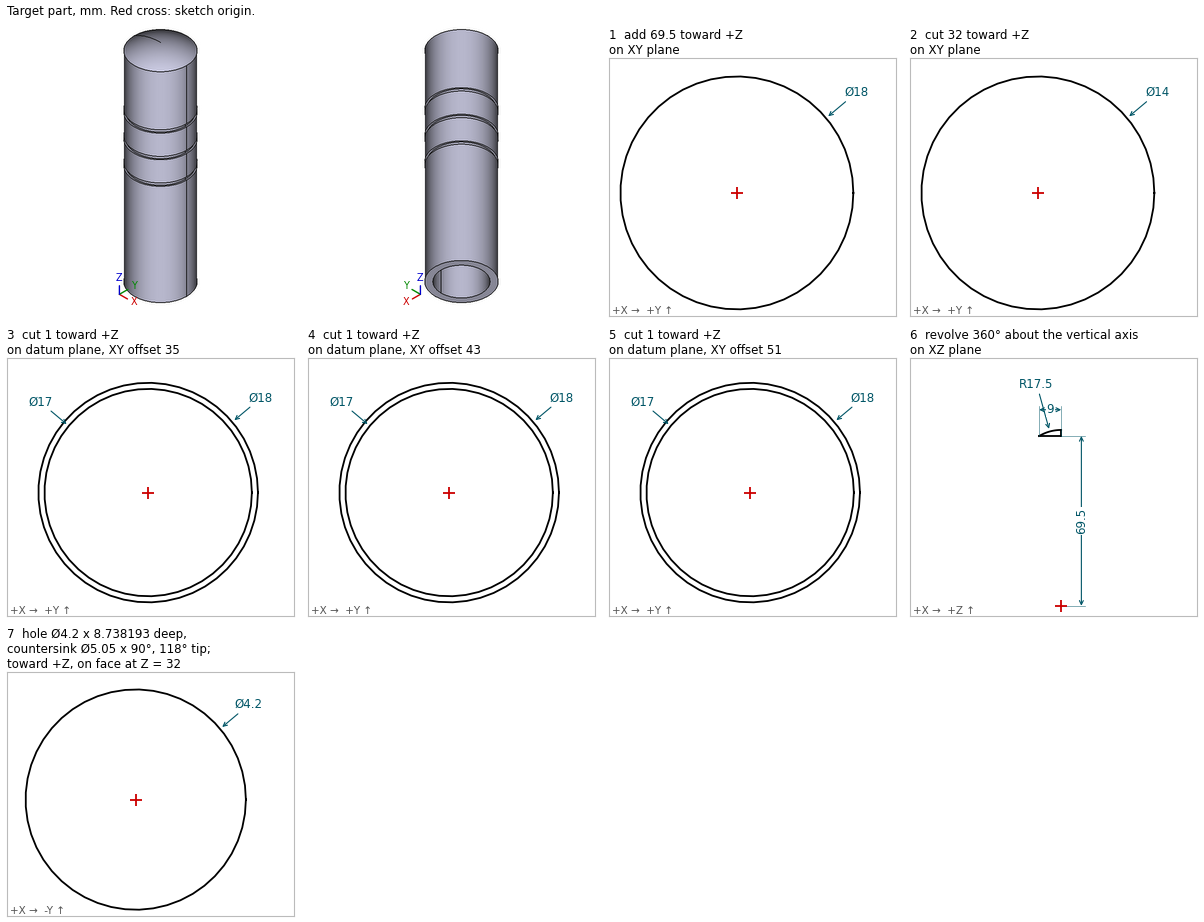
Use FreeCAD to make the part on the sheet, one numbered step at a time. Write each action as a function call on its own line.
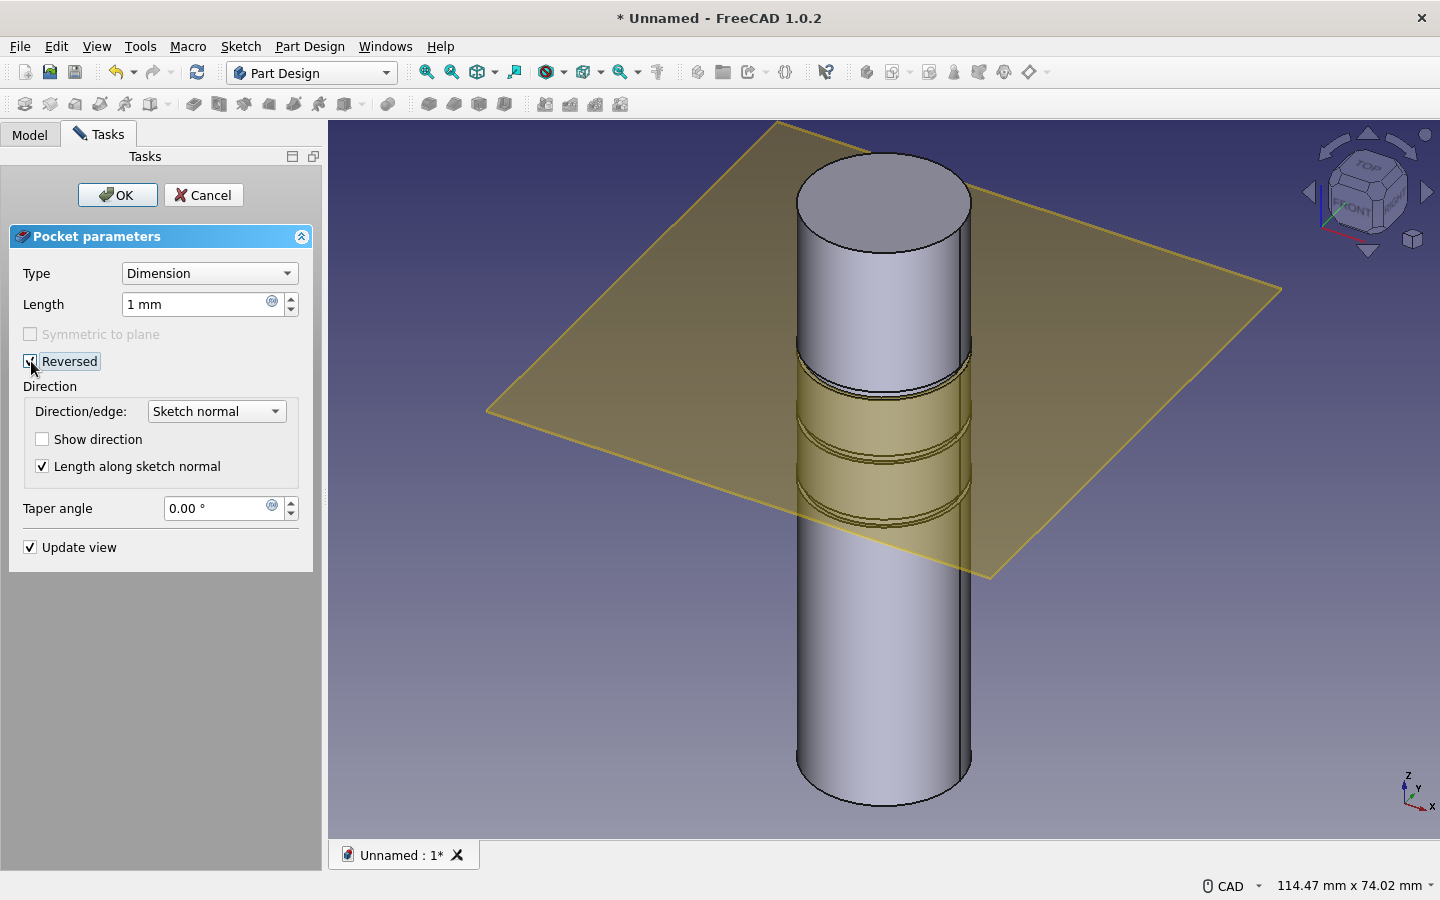
click(118, 195)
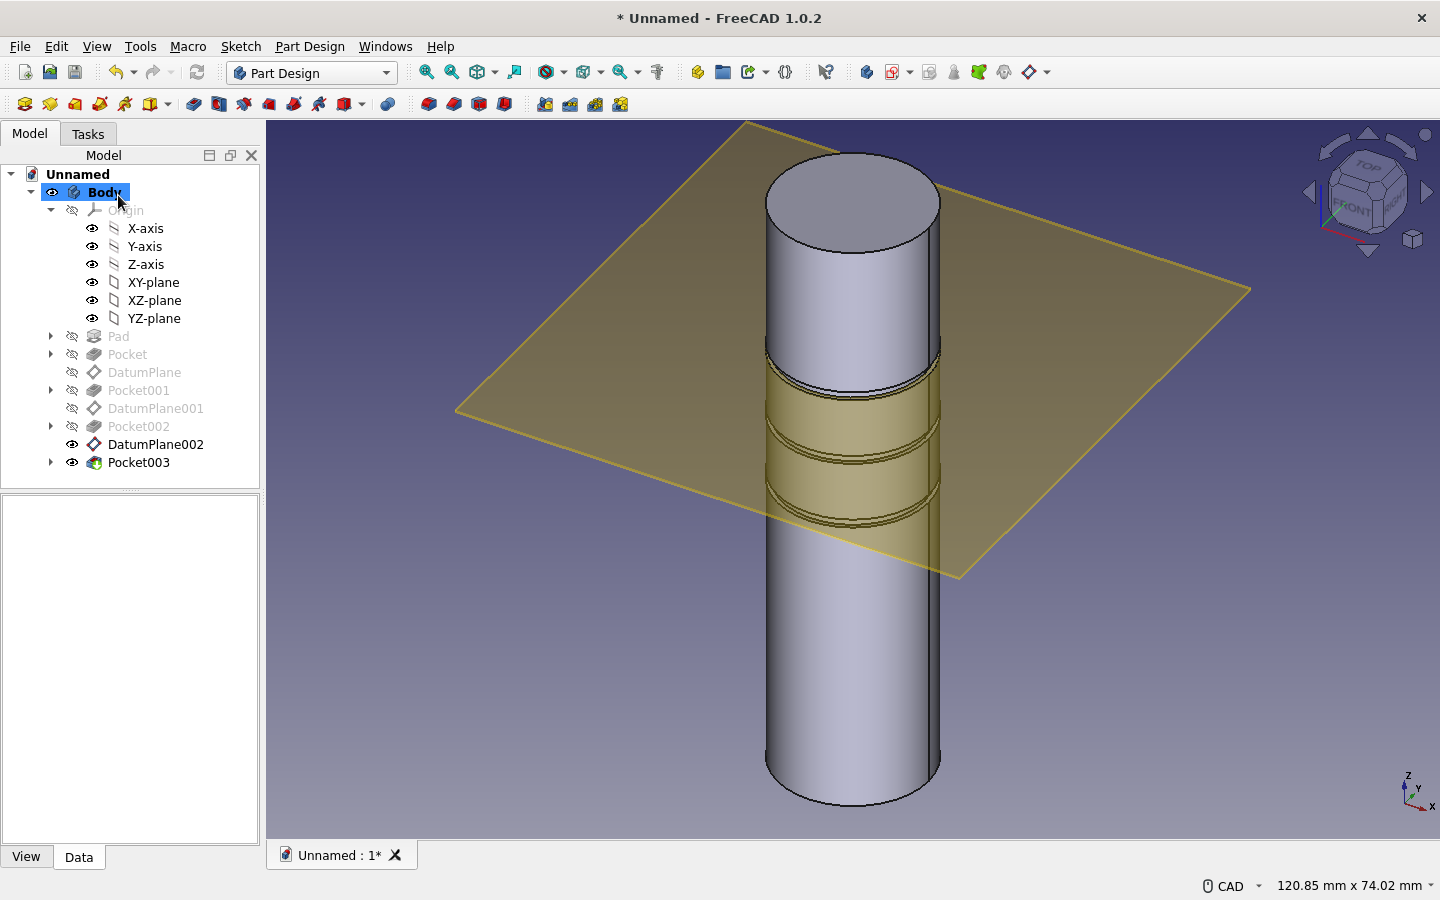
click(117, 444)
key(space)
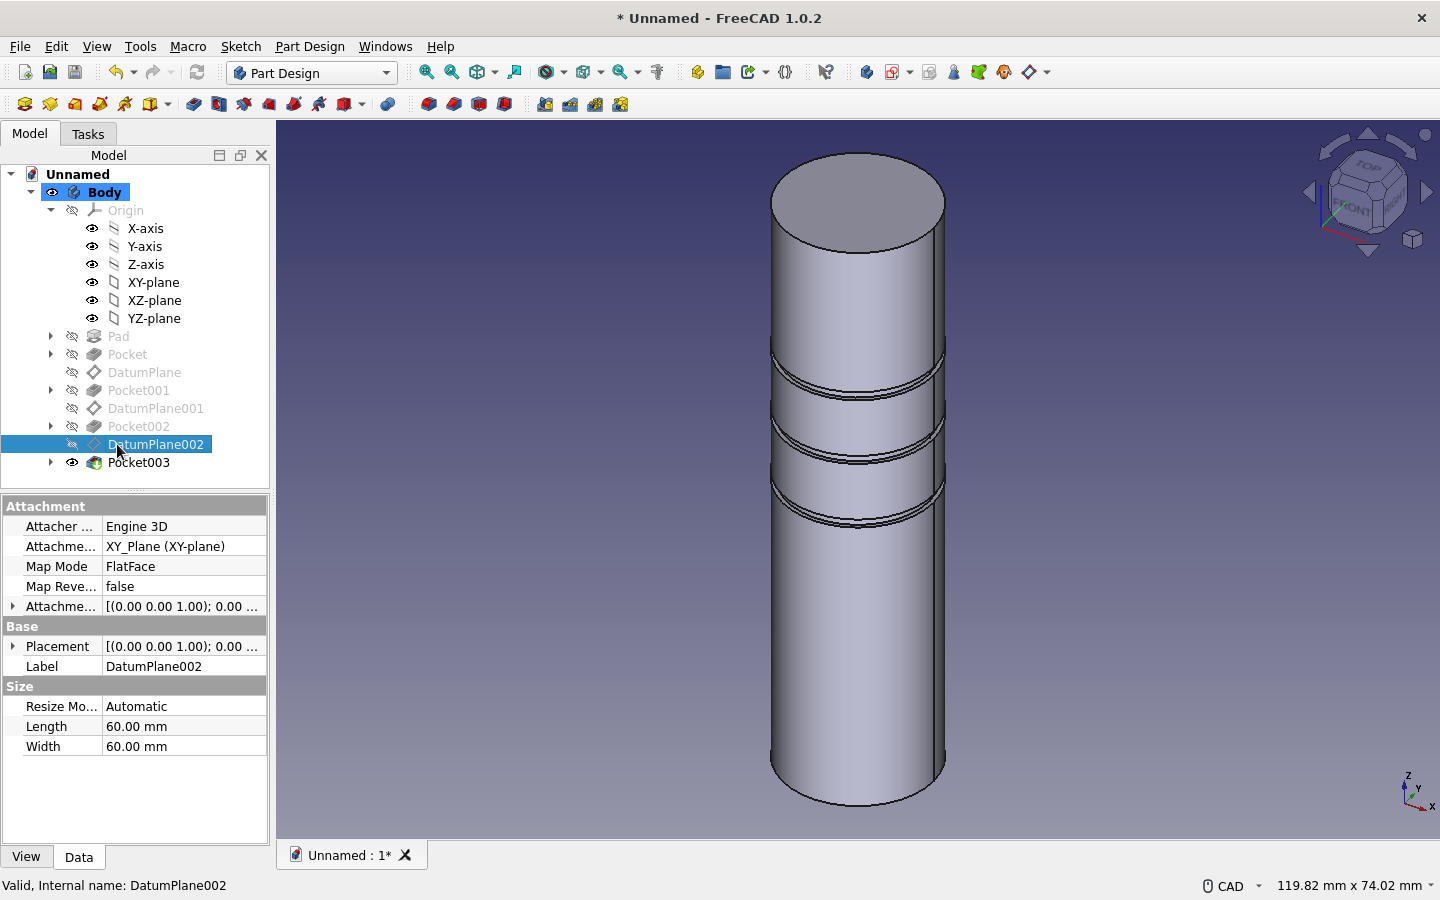
click(316, 799)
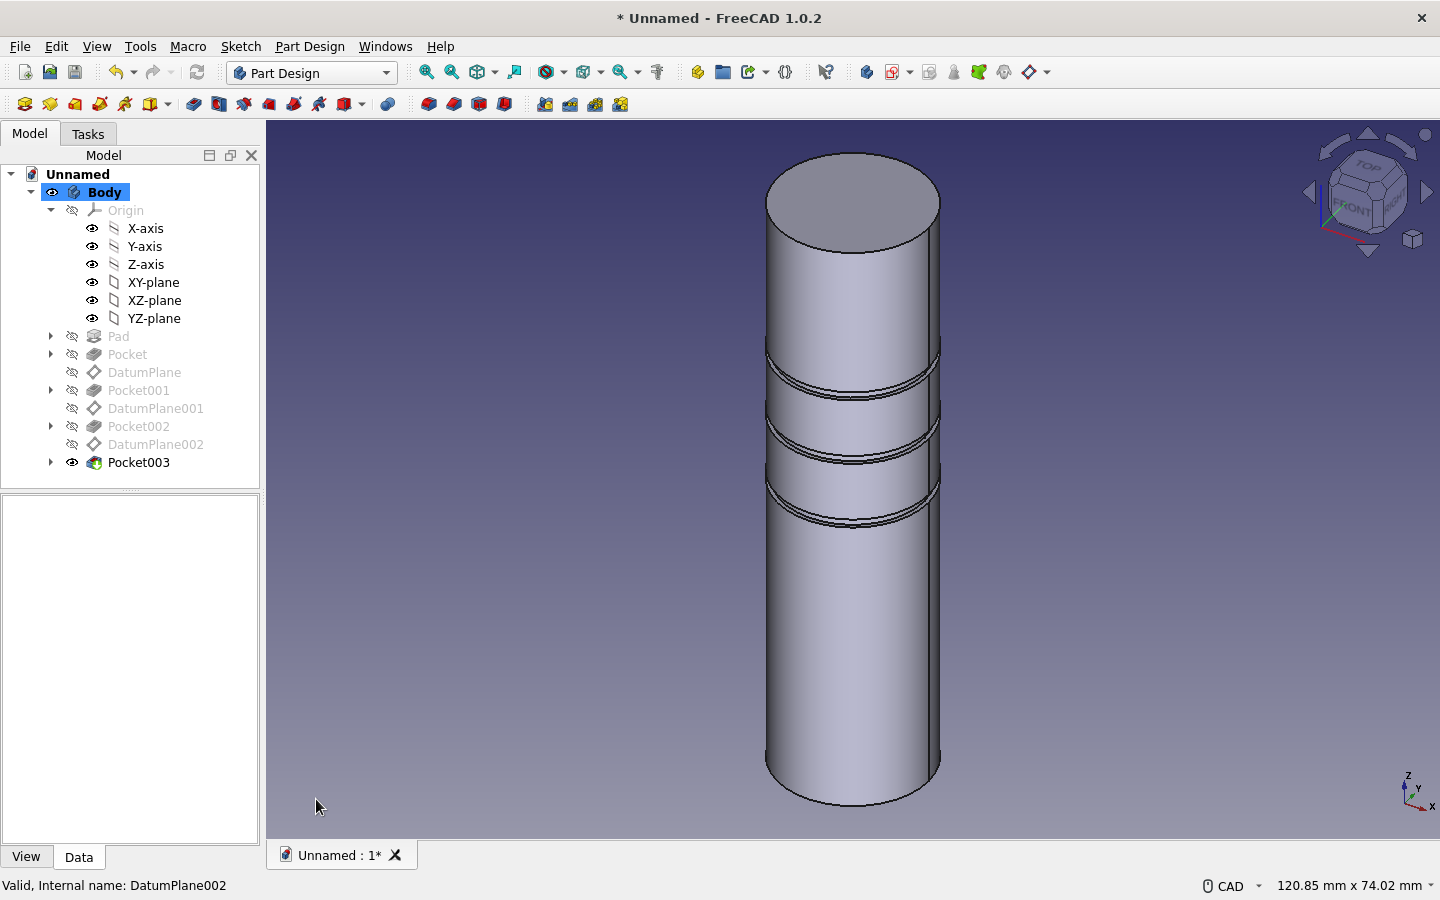
click(892, 72)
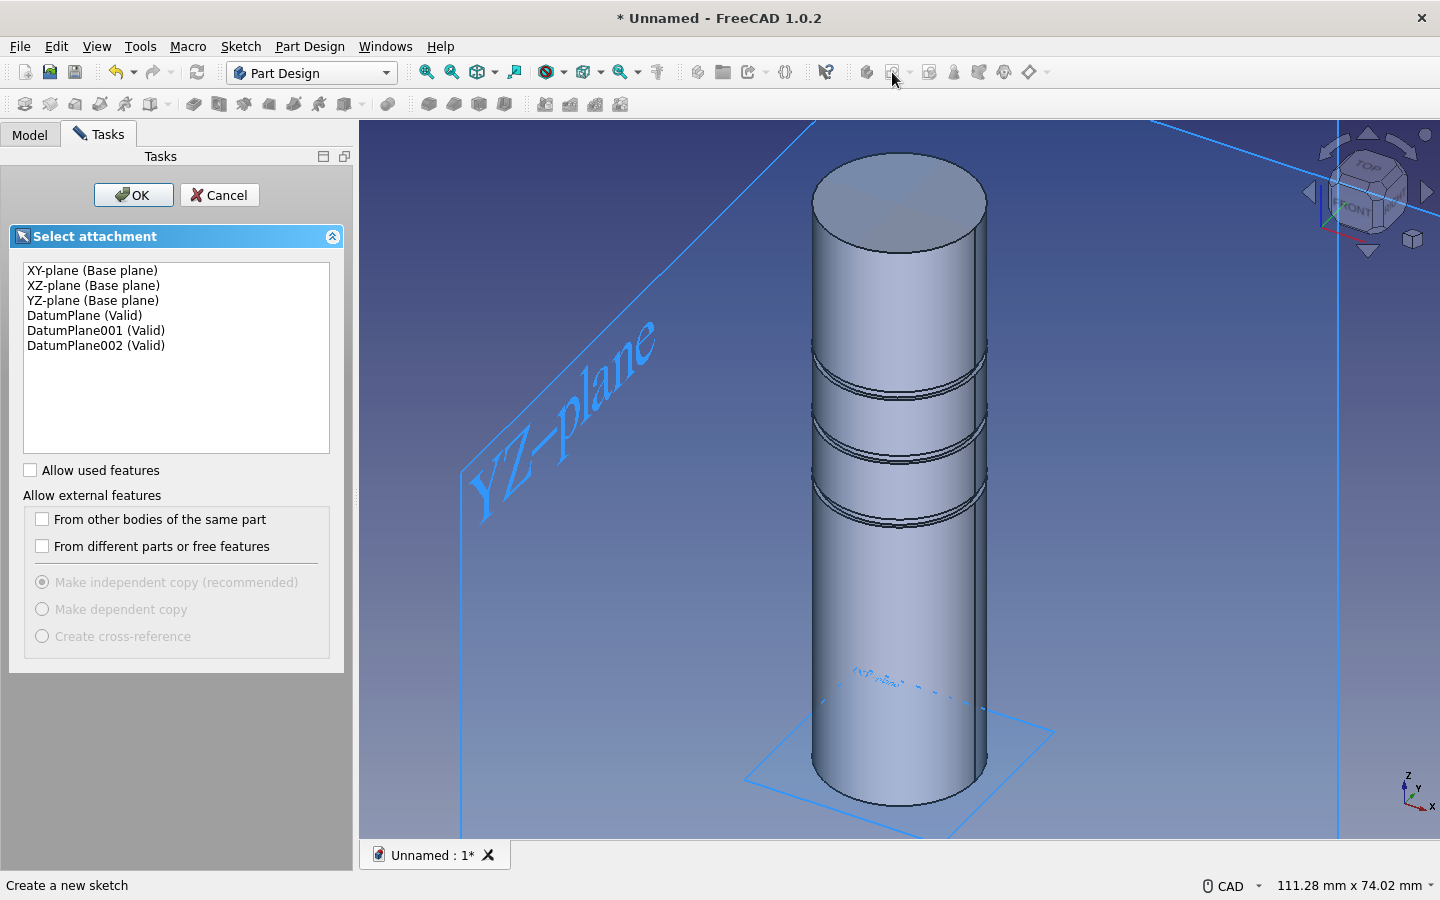
click(84, 286)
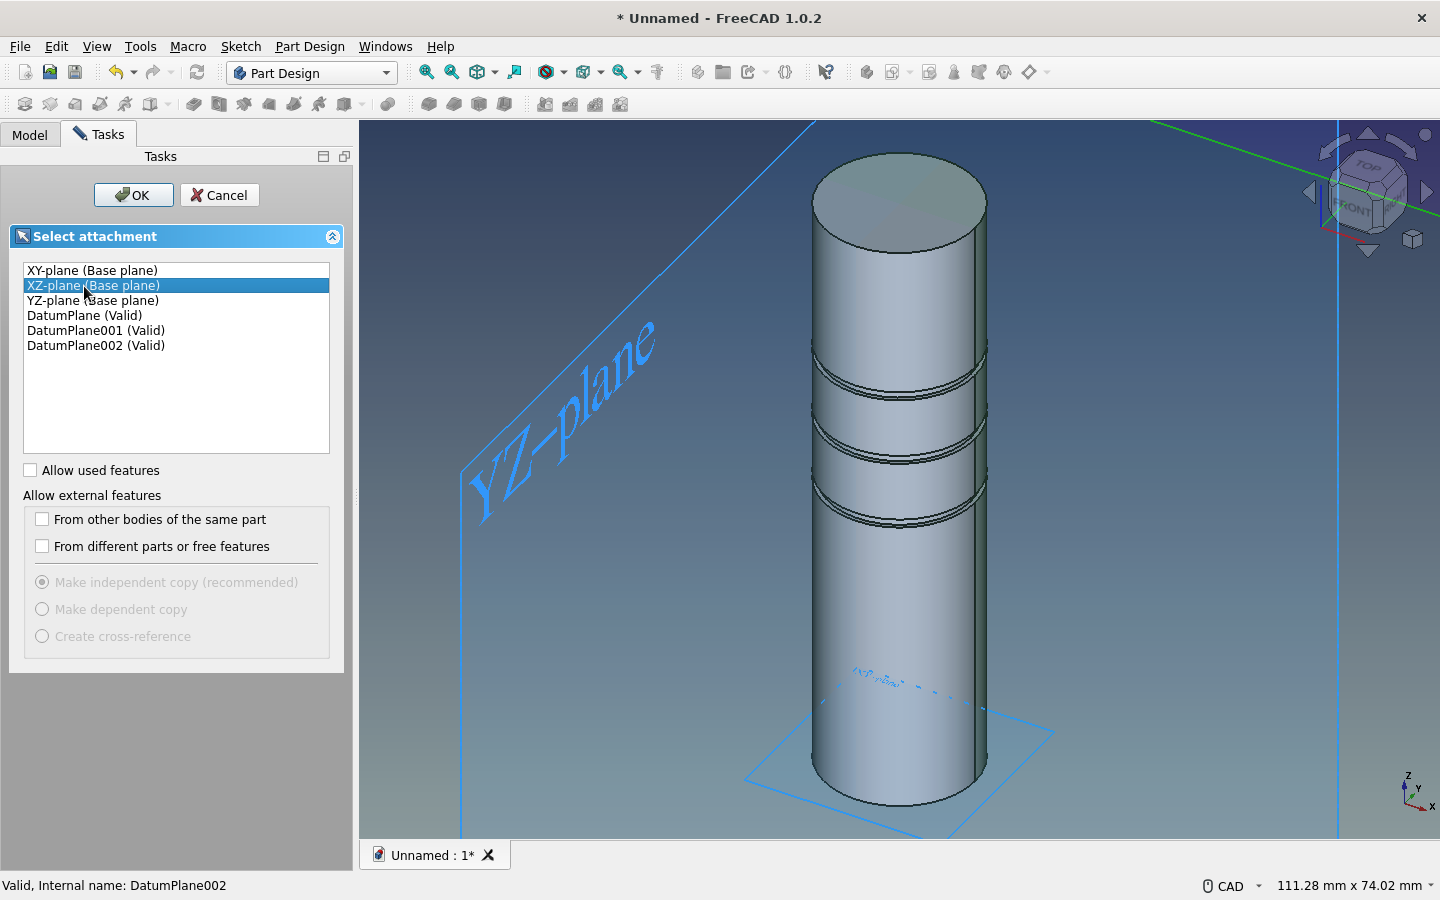
click(134, 195)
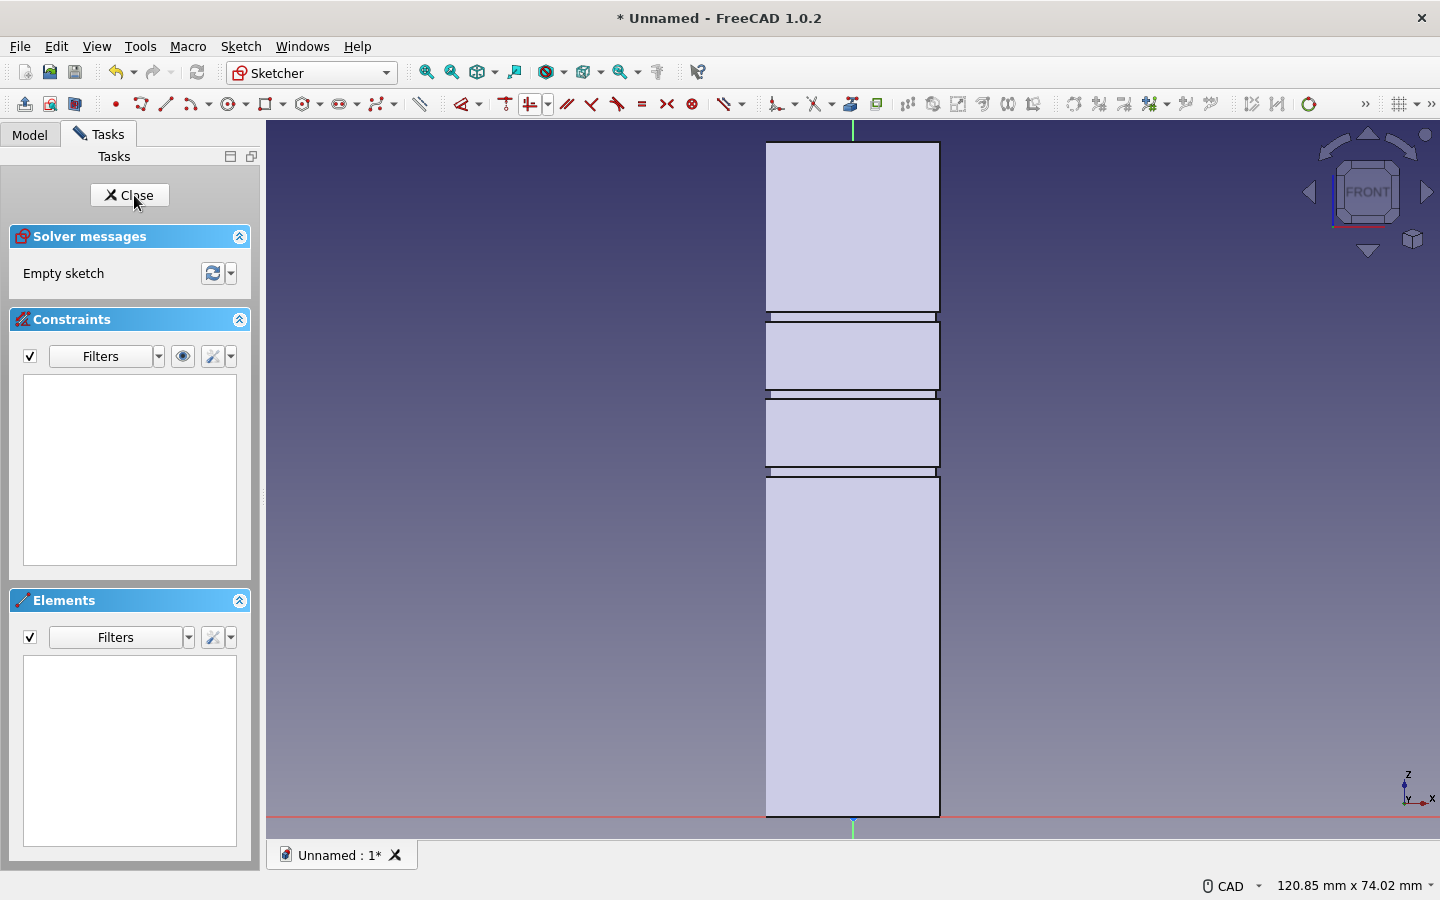
key(q)
key(s)